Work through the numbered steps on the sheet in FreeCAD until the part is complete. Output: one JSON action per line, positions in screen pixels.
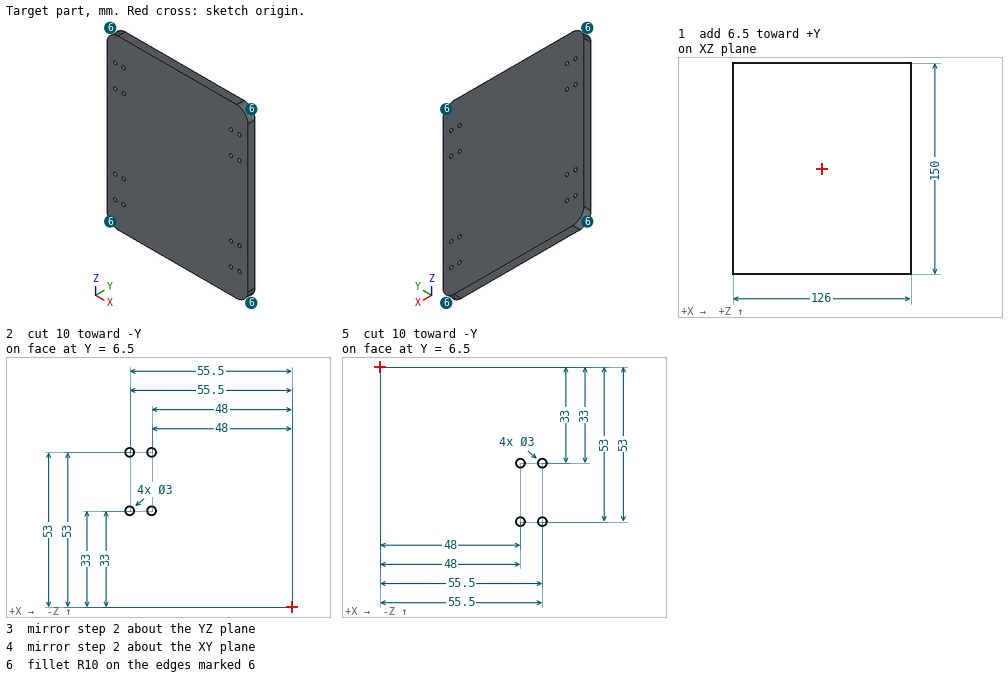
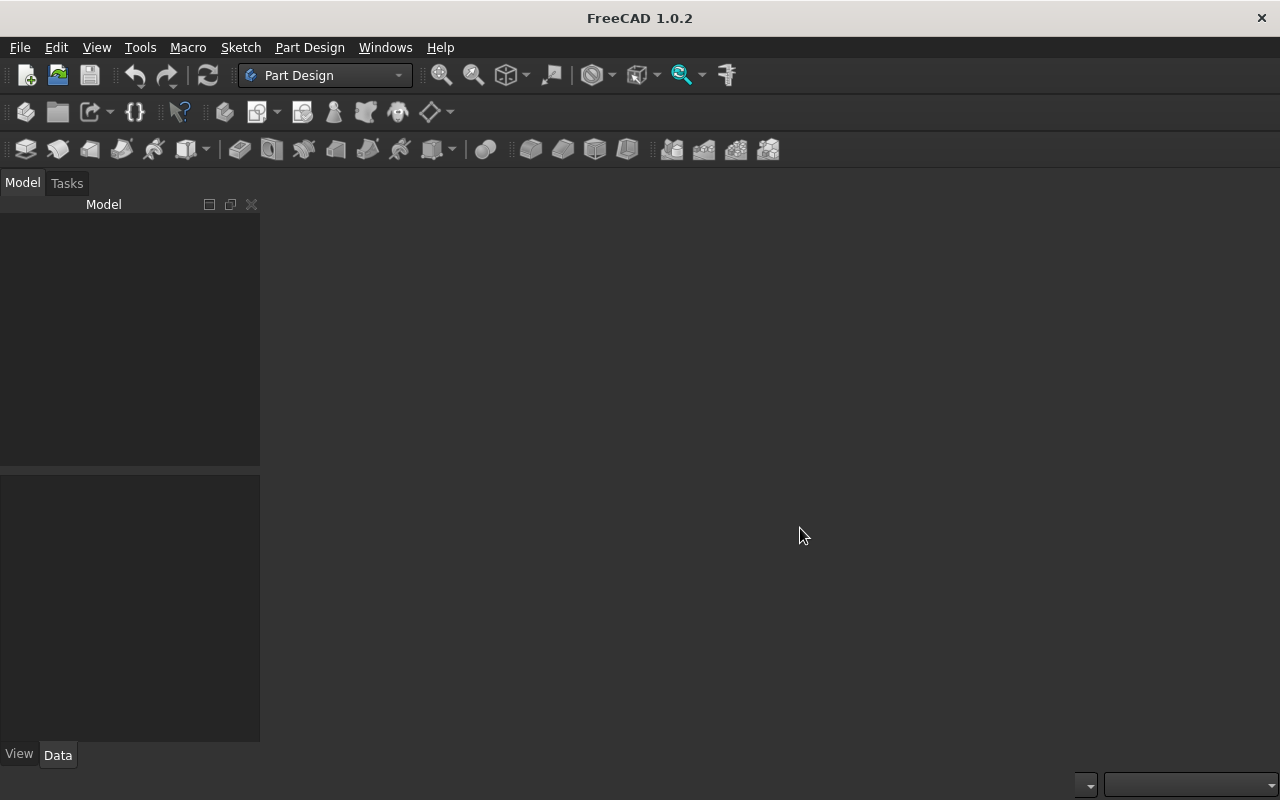
{"action": "key", "text": "ctrl+n"}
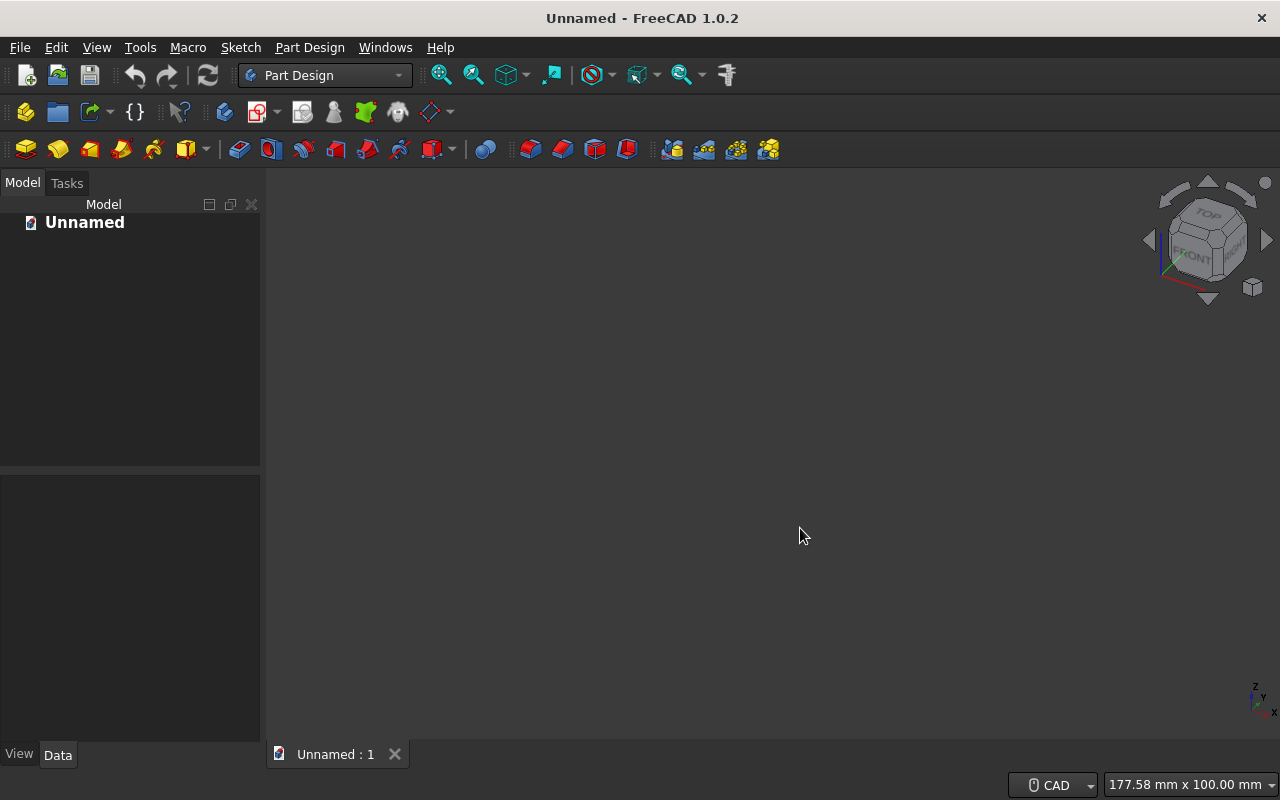
{"action": "left_click", "coordinate": [258, 112]}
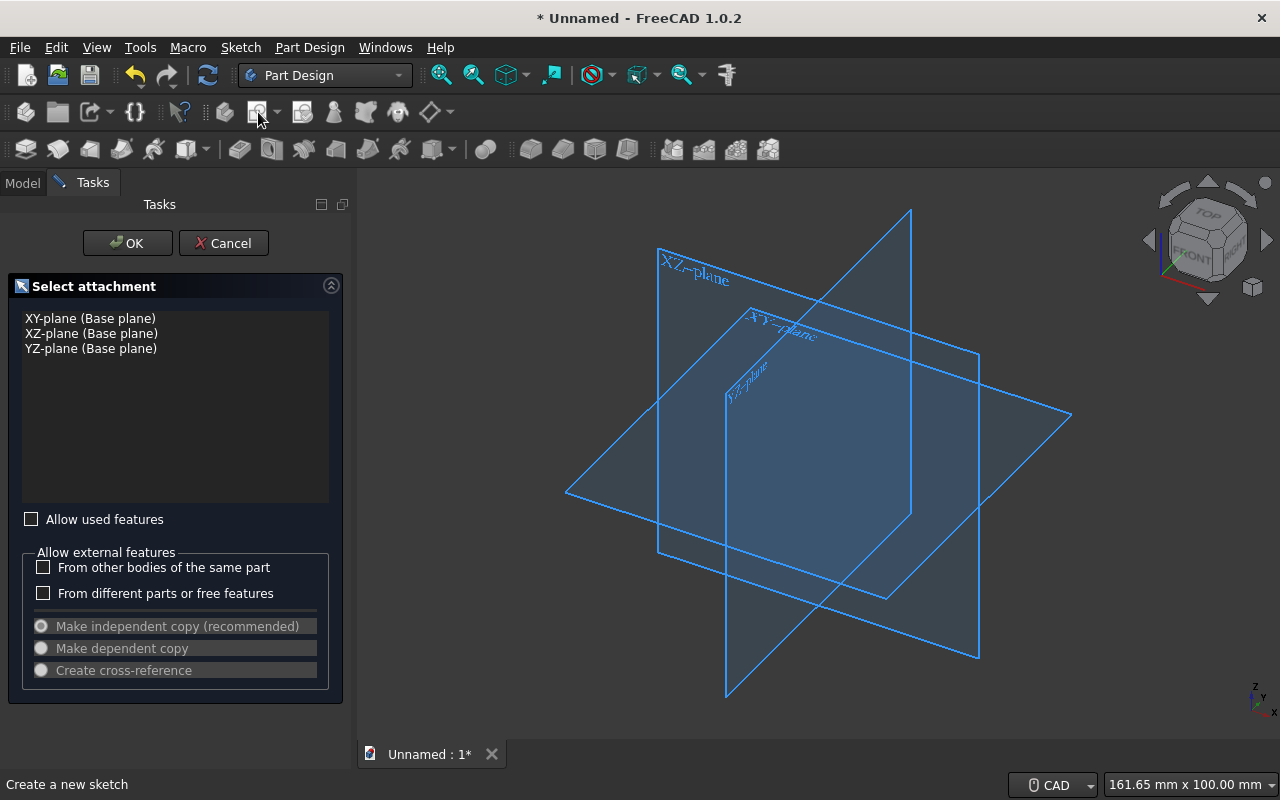
{"action": "left_click", "coordinate": [82, 334]}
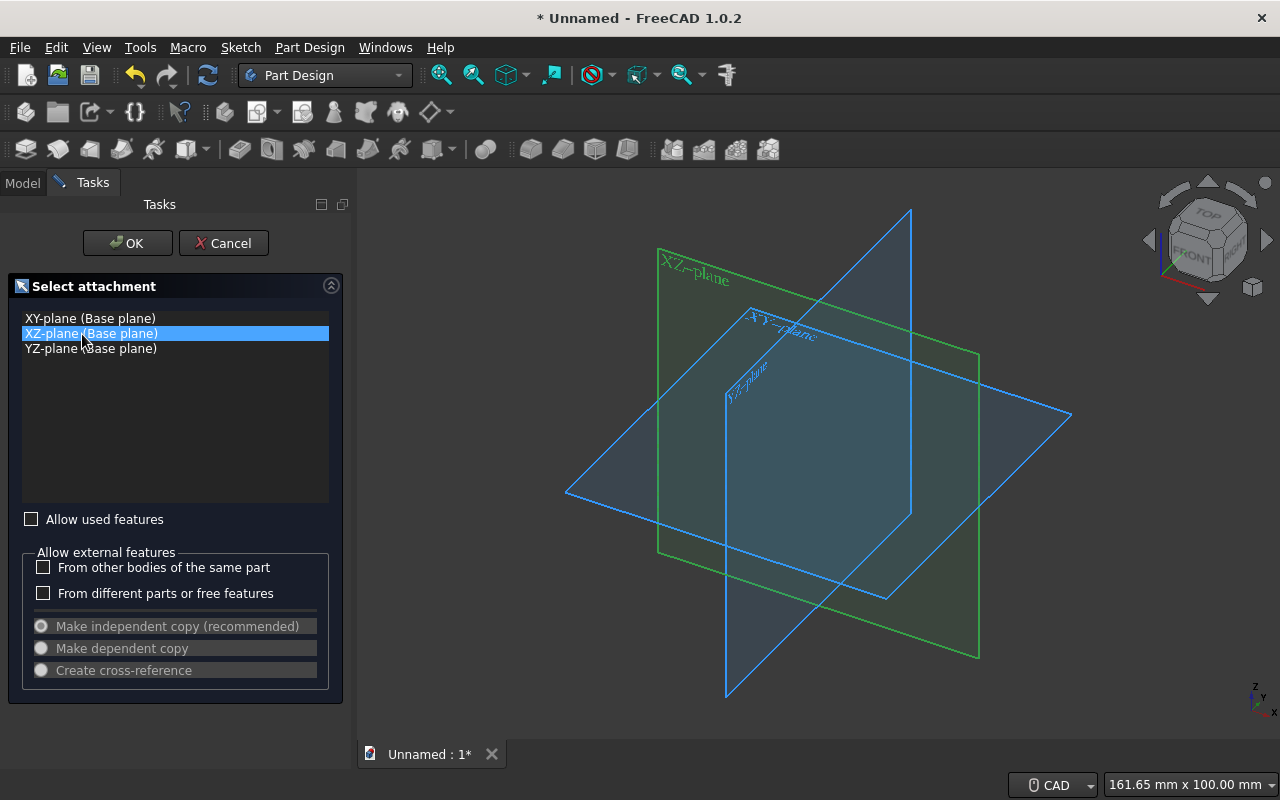
{"action": "left_click", "coordinate": [128, 243]}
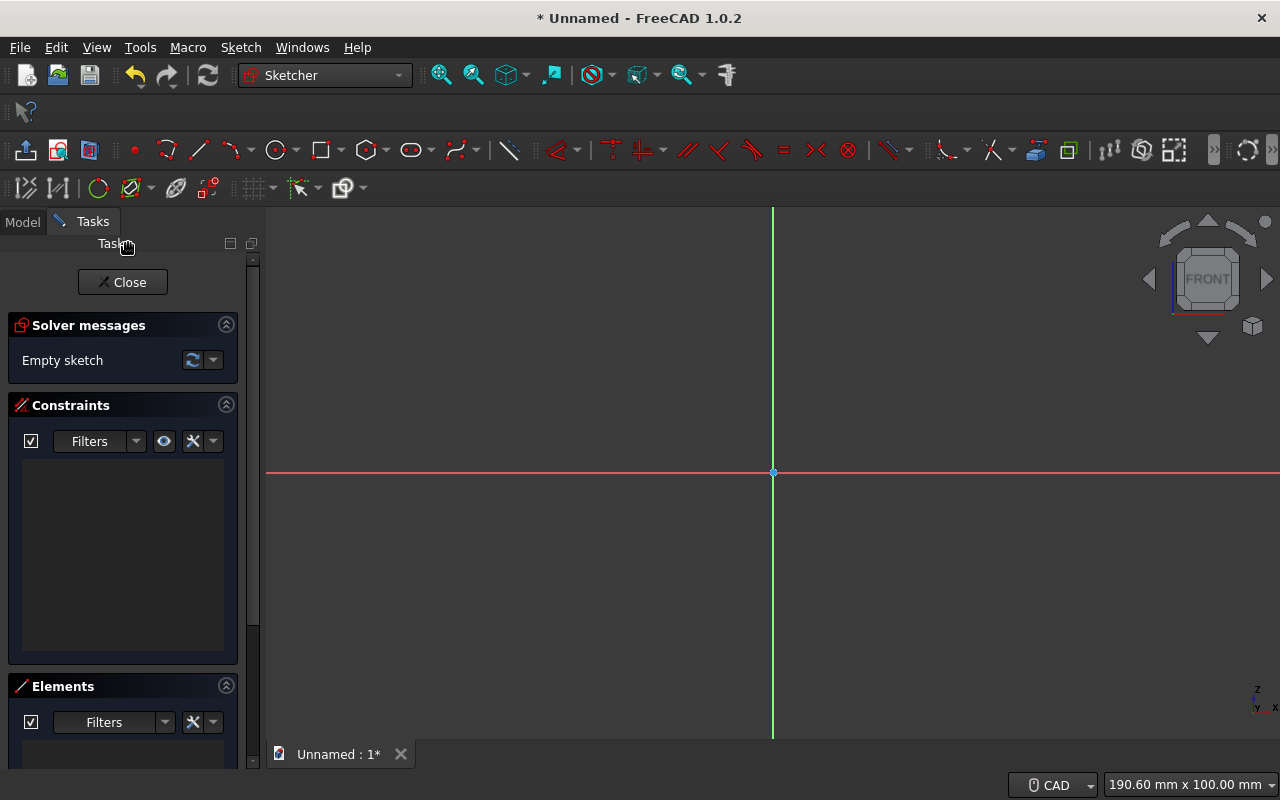
{"action": "scroll", "coordinate": [649, 473], "scroll_direction": "down", "scroll_amount": 4}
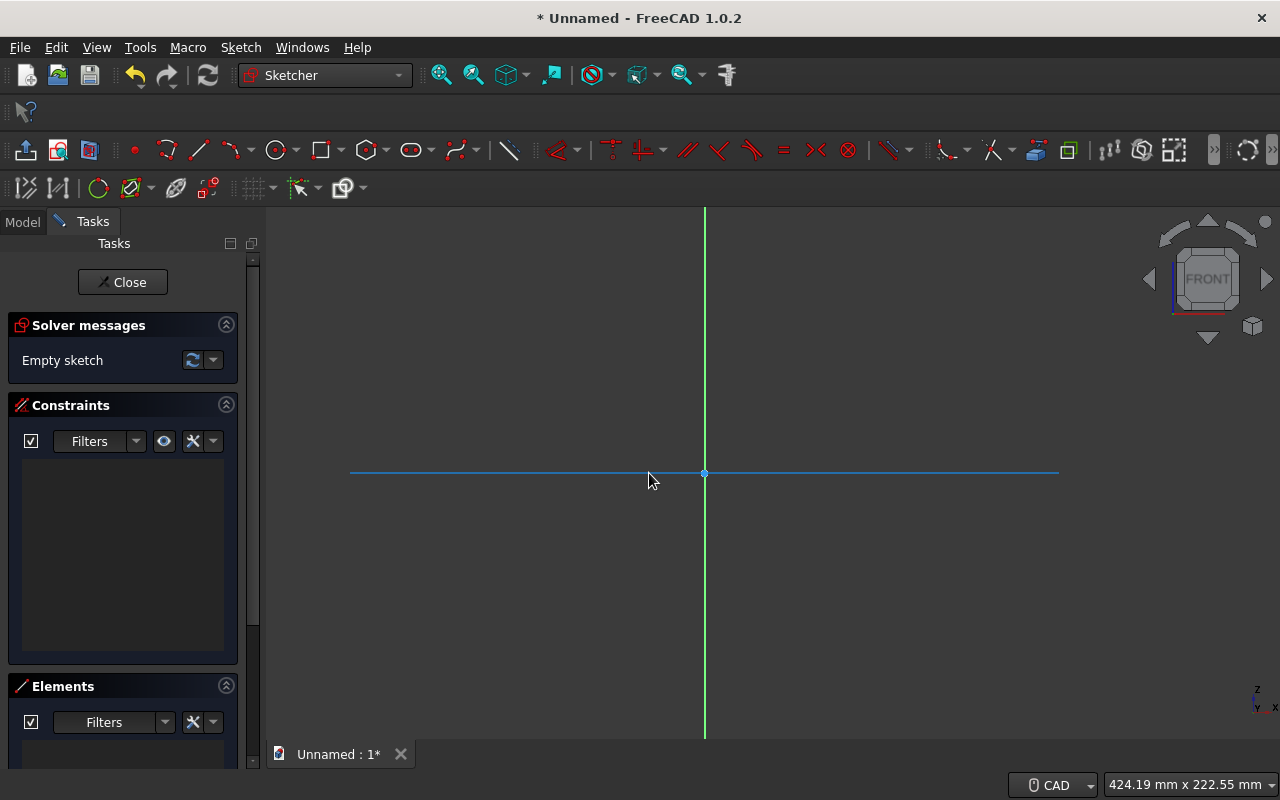
{"action": "left_click", "coordinate": [344, 150]}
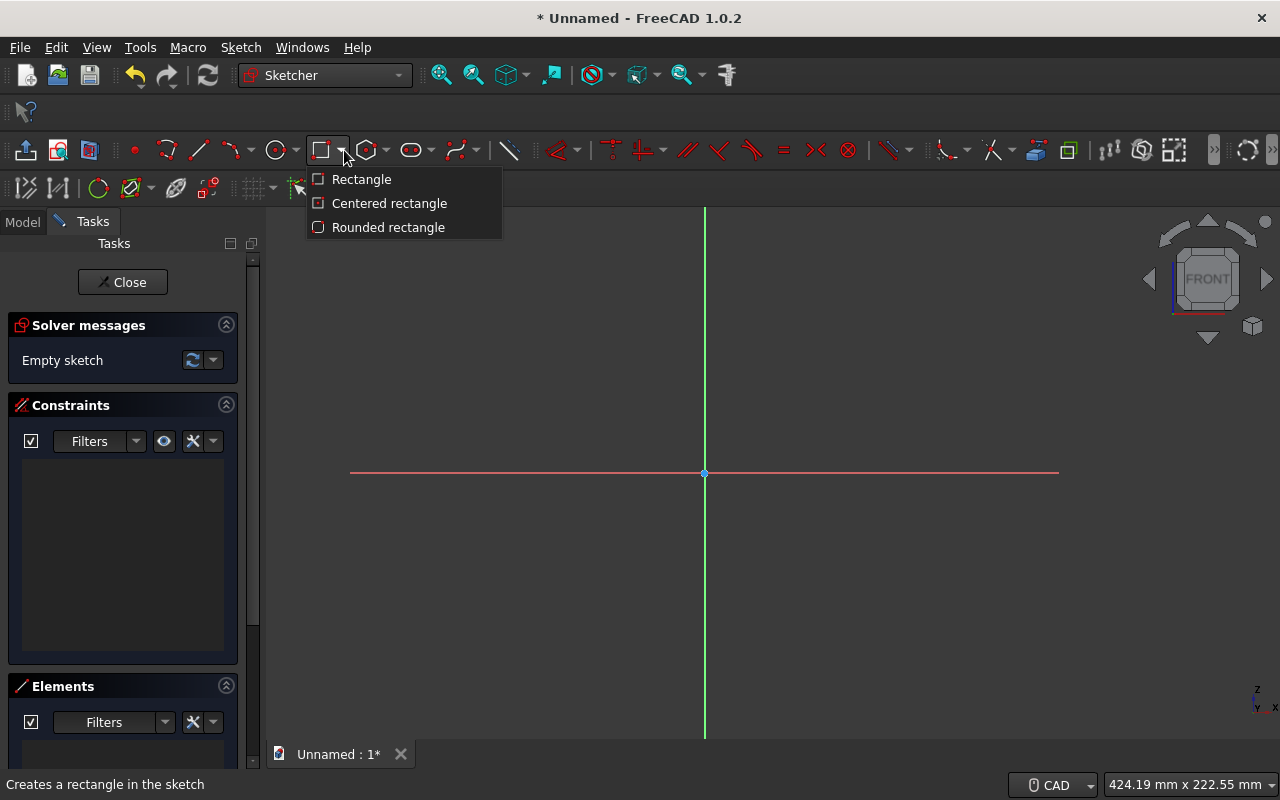
{"action": "left_click", "coordinate": [404, 203]}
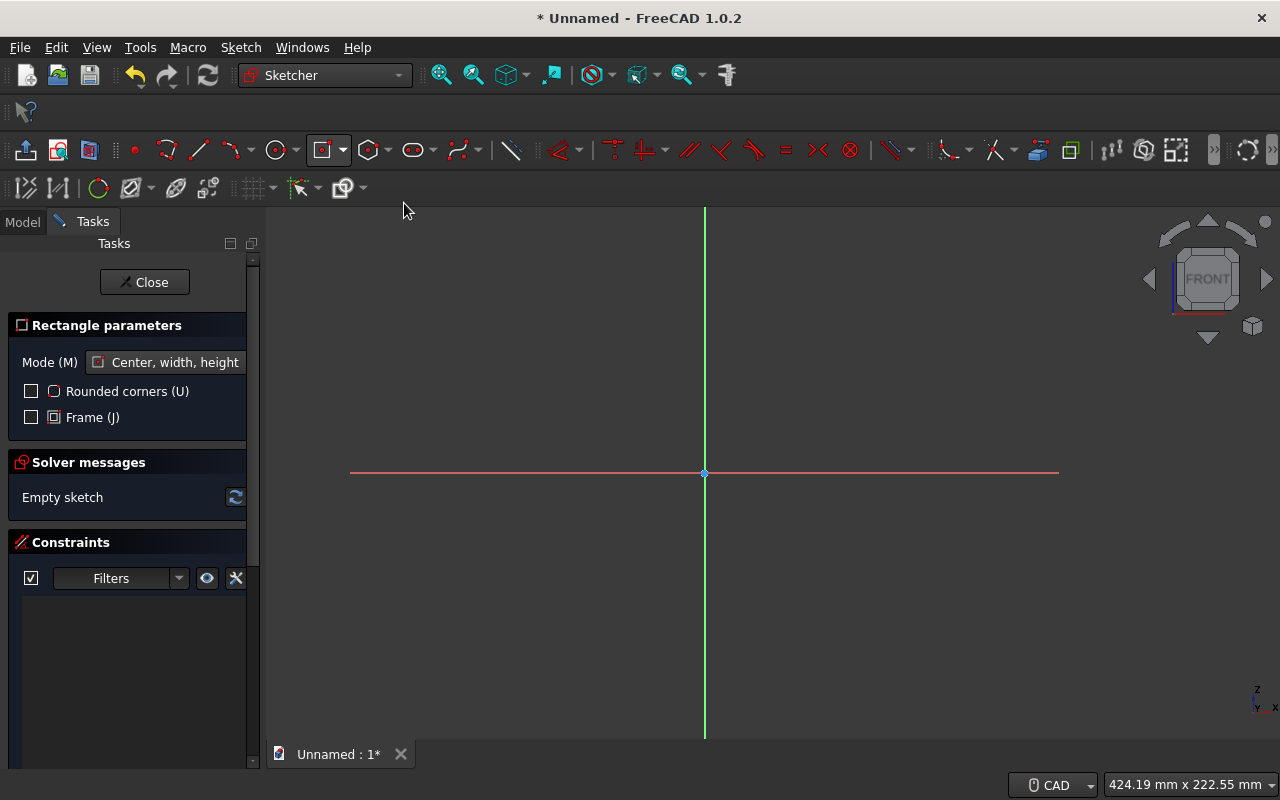
{"action": "left_click", "coordinate": [705, 473]}
{"action": "left_click", "coordinate": [856, 294]}
{"action": "key", "text": "Escape"}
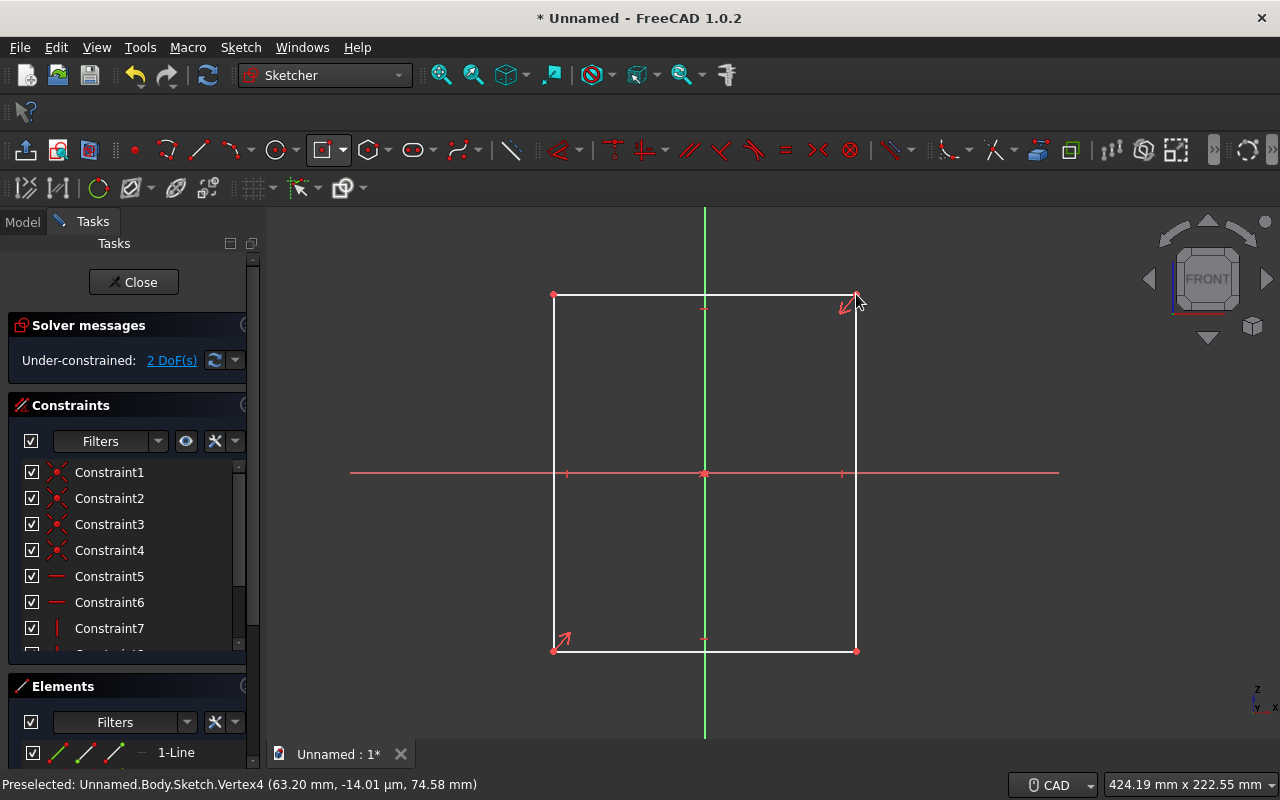
{"action": "left_click", "coordinate": [558, 150]}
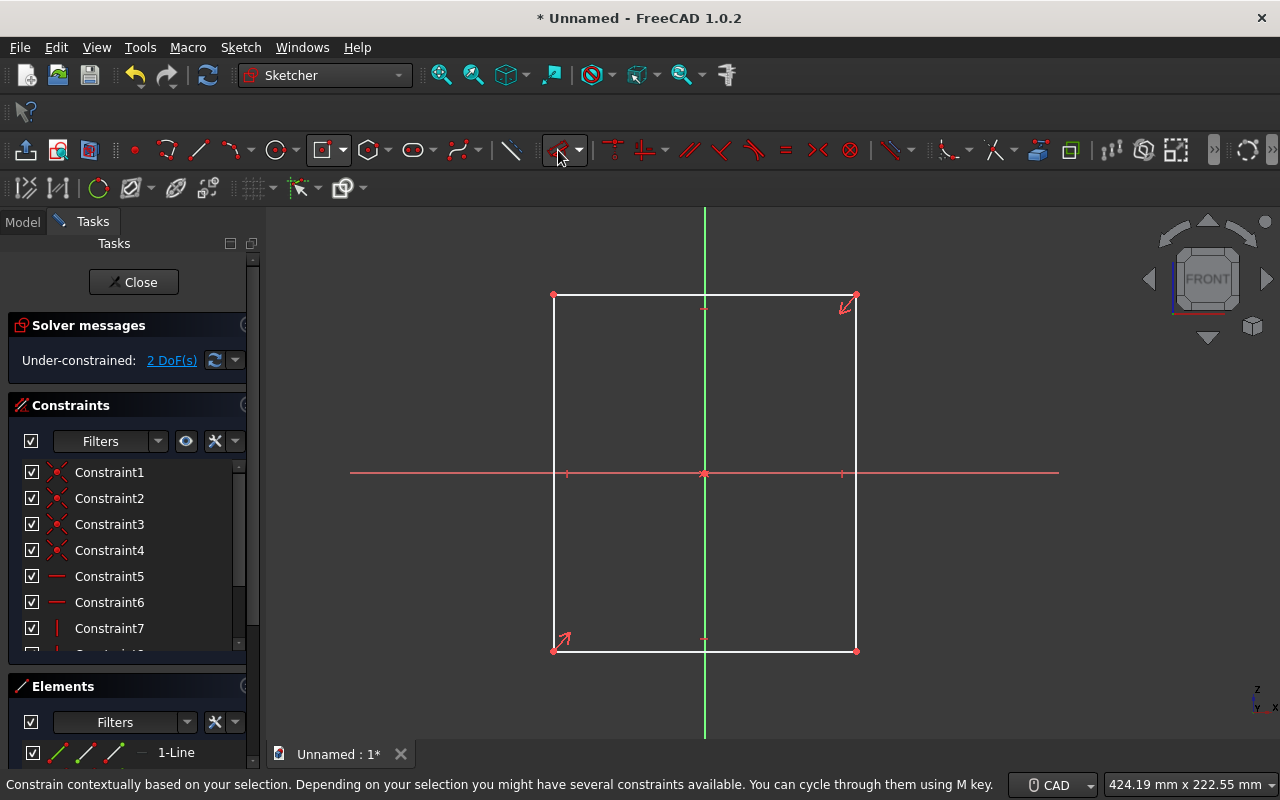
{"action": "left_click", "coordinate": [644, 652]}
{"action": "left_click", "coordinate": [635, 686]}